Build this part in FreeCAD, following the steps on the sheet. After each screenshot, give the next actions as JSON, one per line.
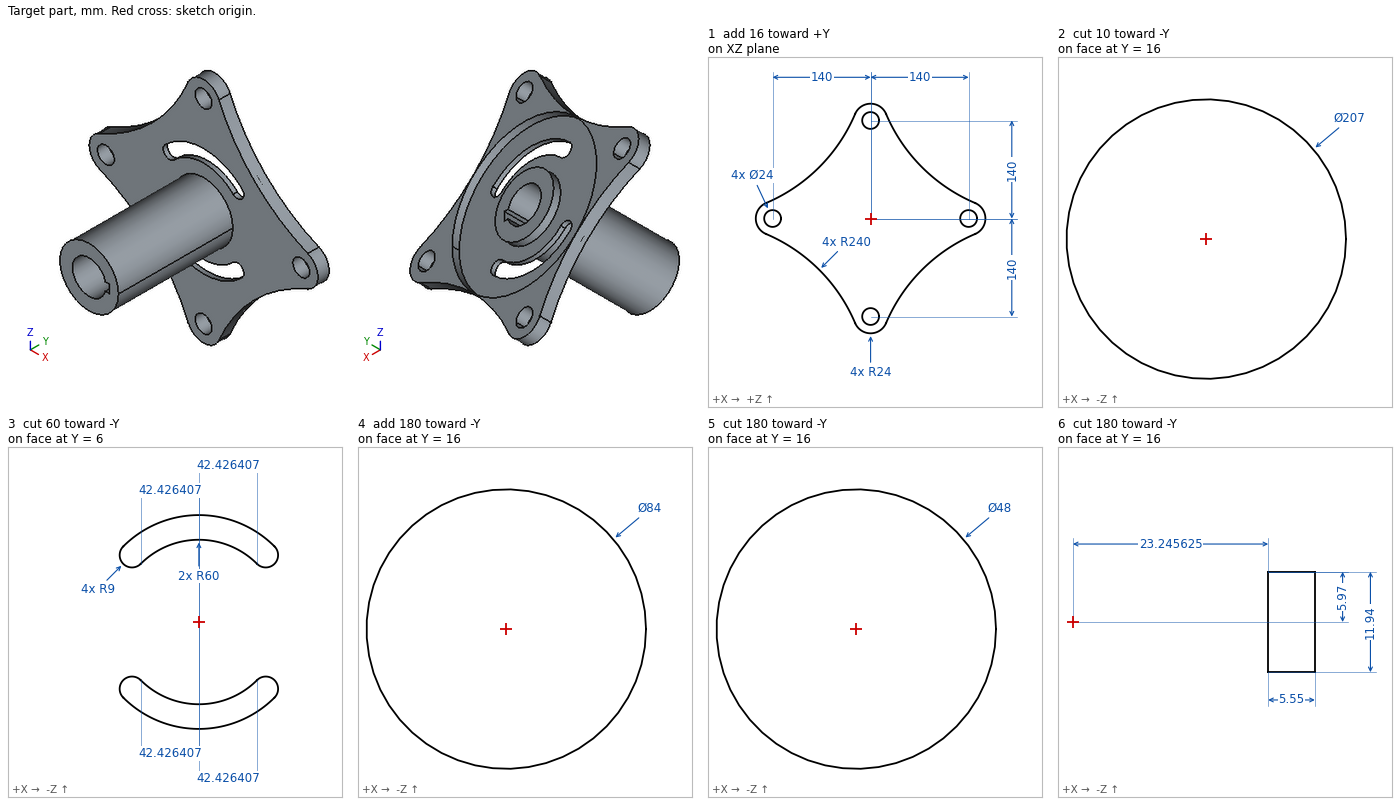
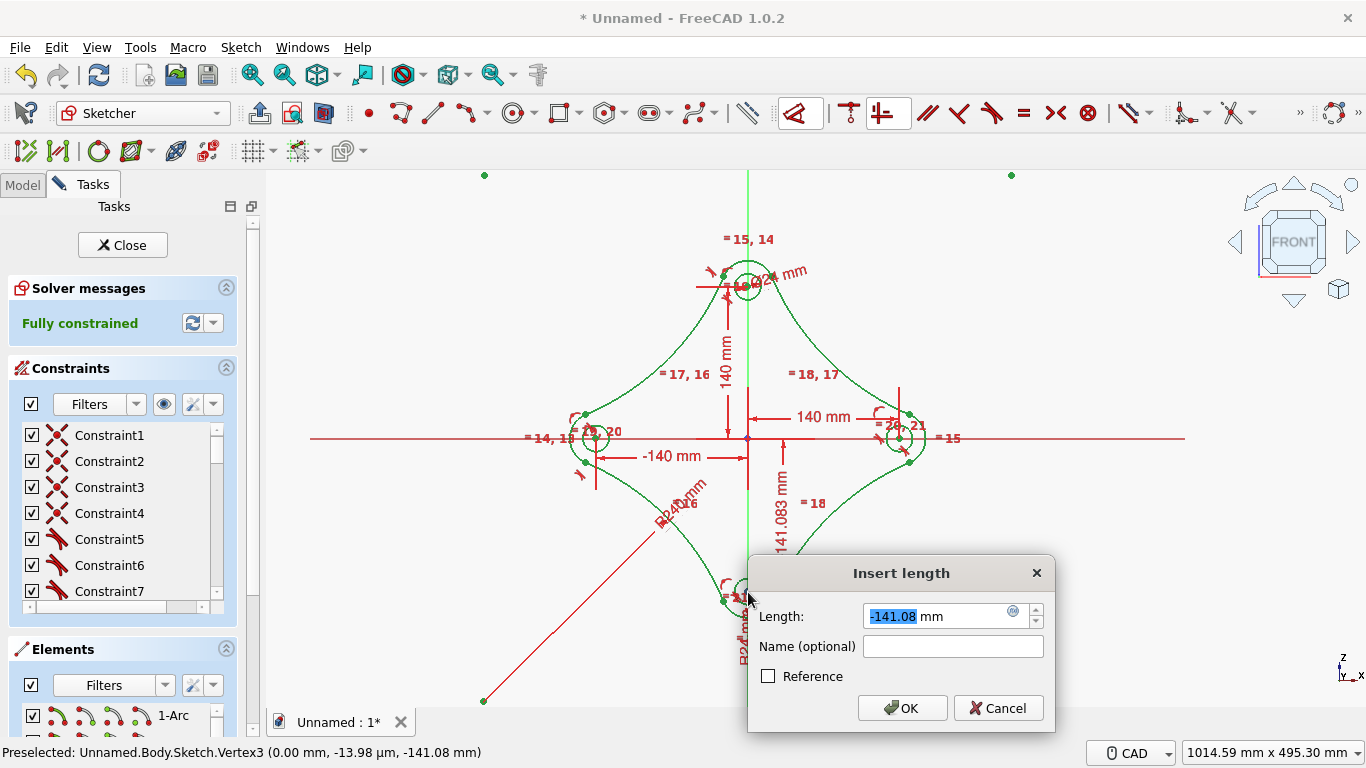
{"action": "type", "text": "-140"}
{"action": "key", "text": "Return"}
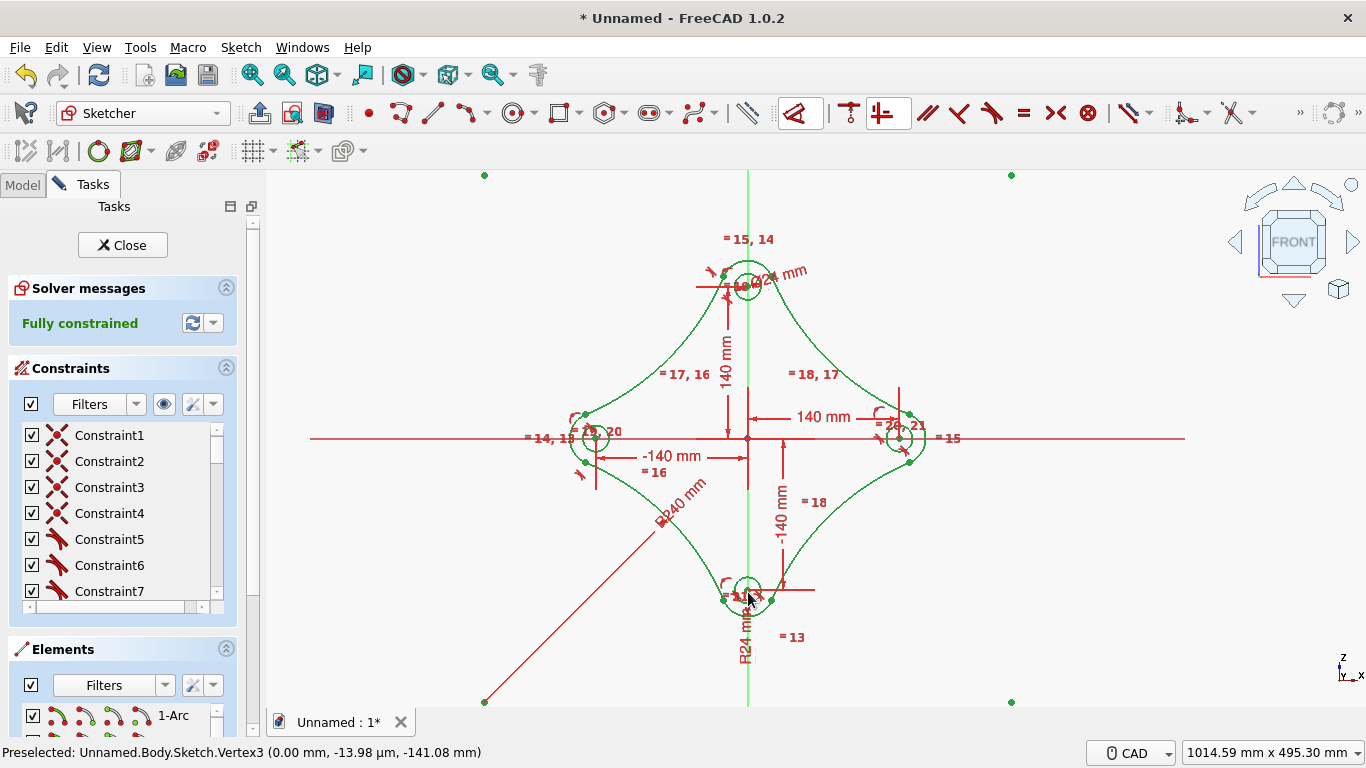
{"action": "left_click", "coordinate": [123, 245]}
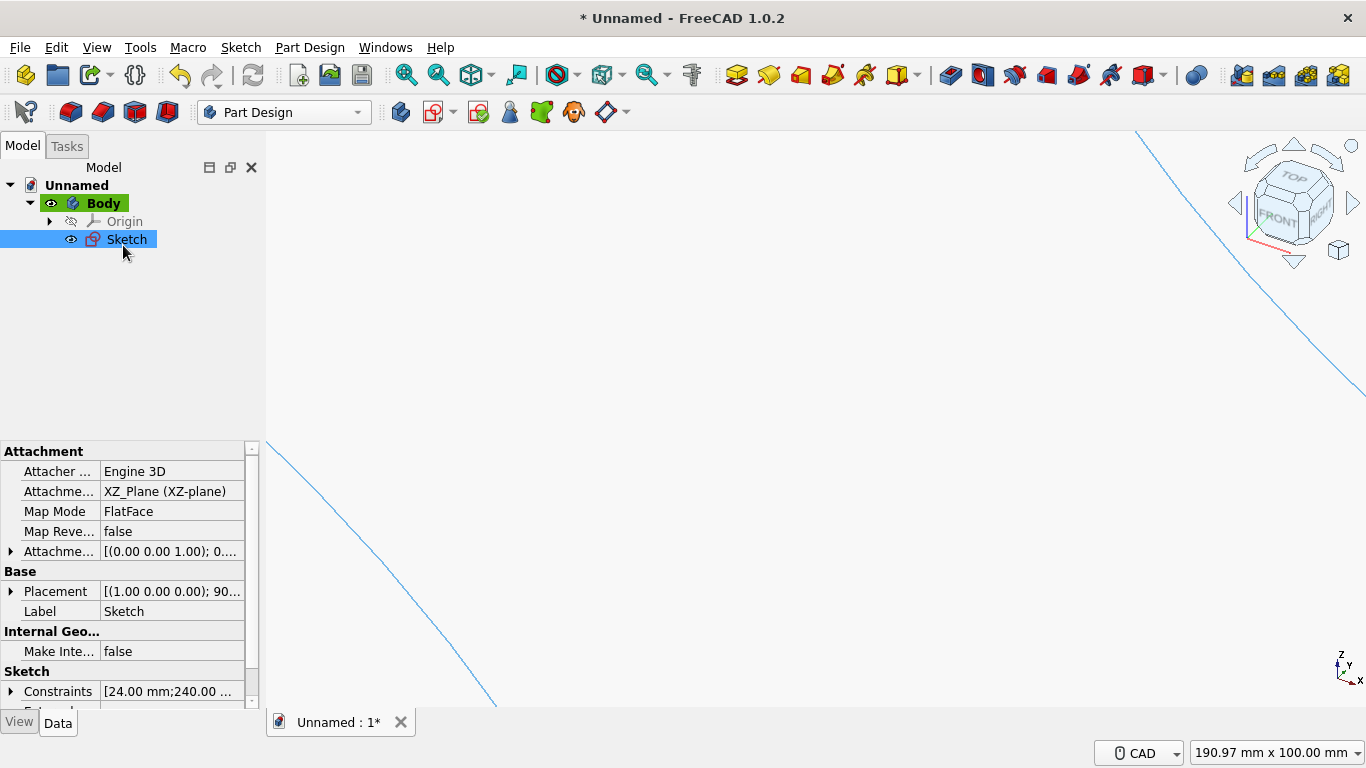
{"action": "left_click", "coordinate": [738, 76]}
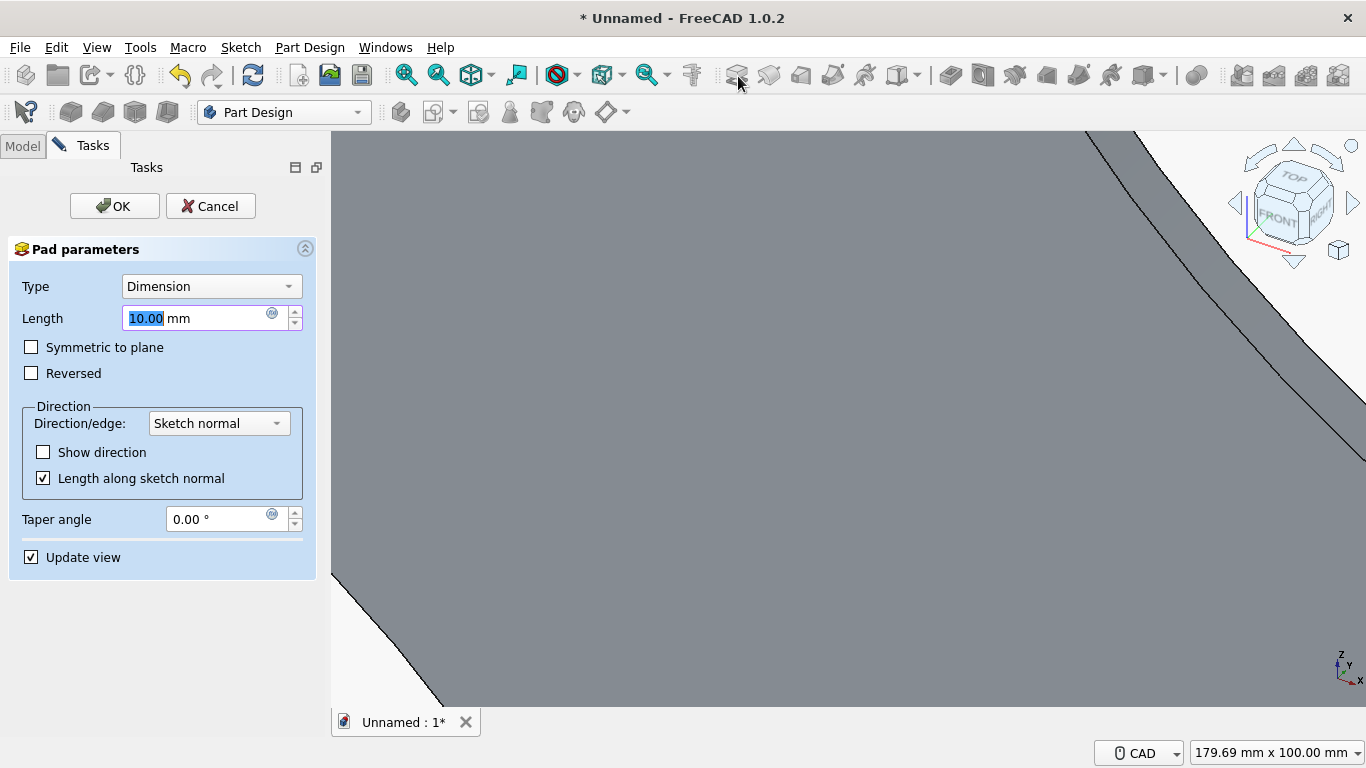
{"action": "type", "text": "16"}
{"action": "key", "text": "Tab"}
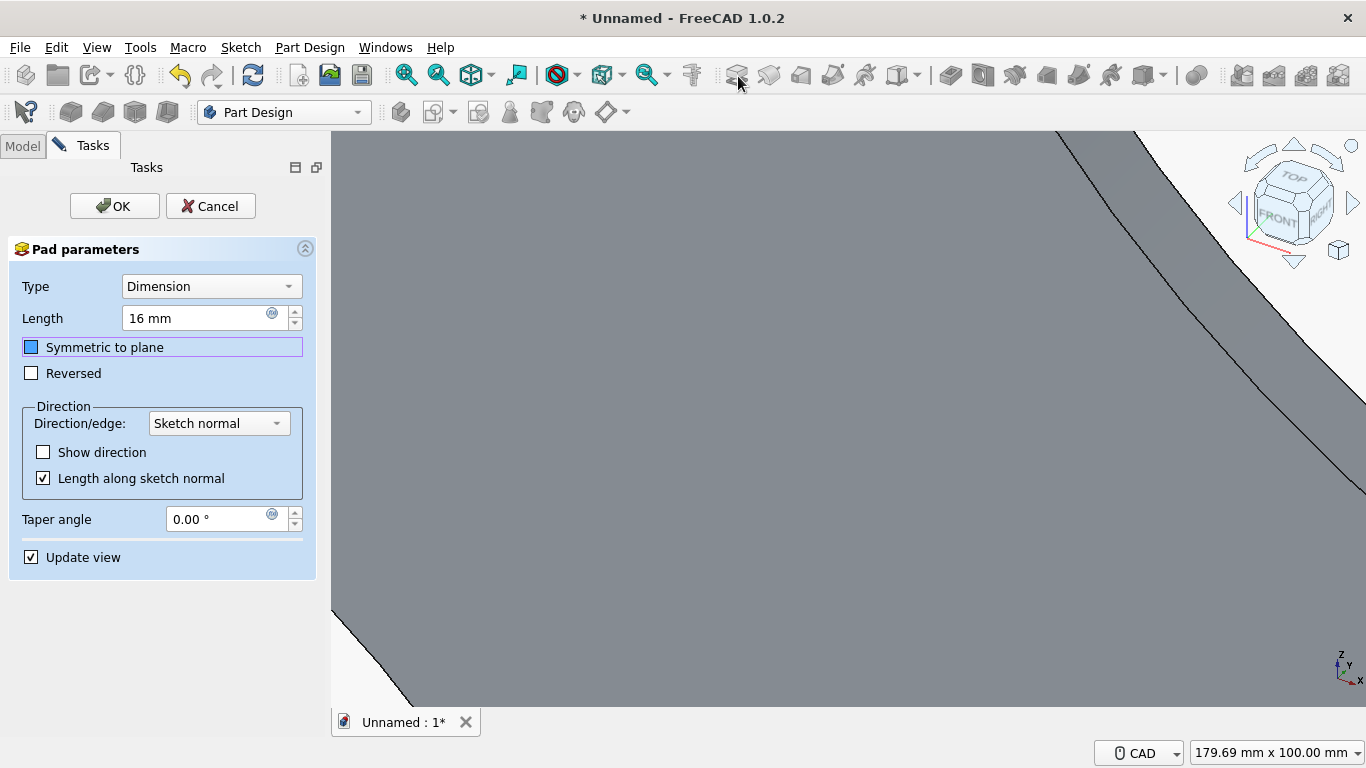
{"action": "left_click", "coordinate": [30, 373]}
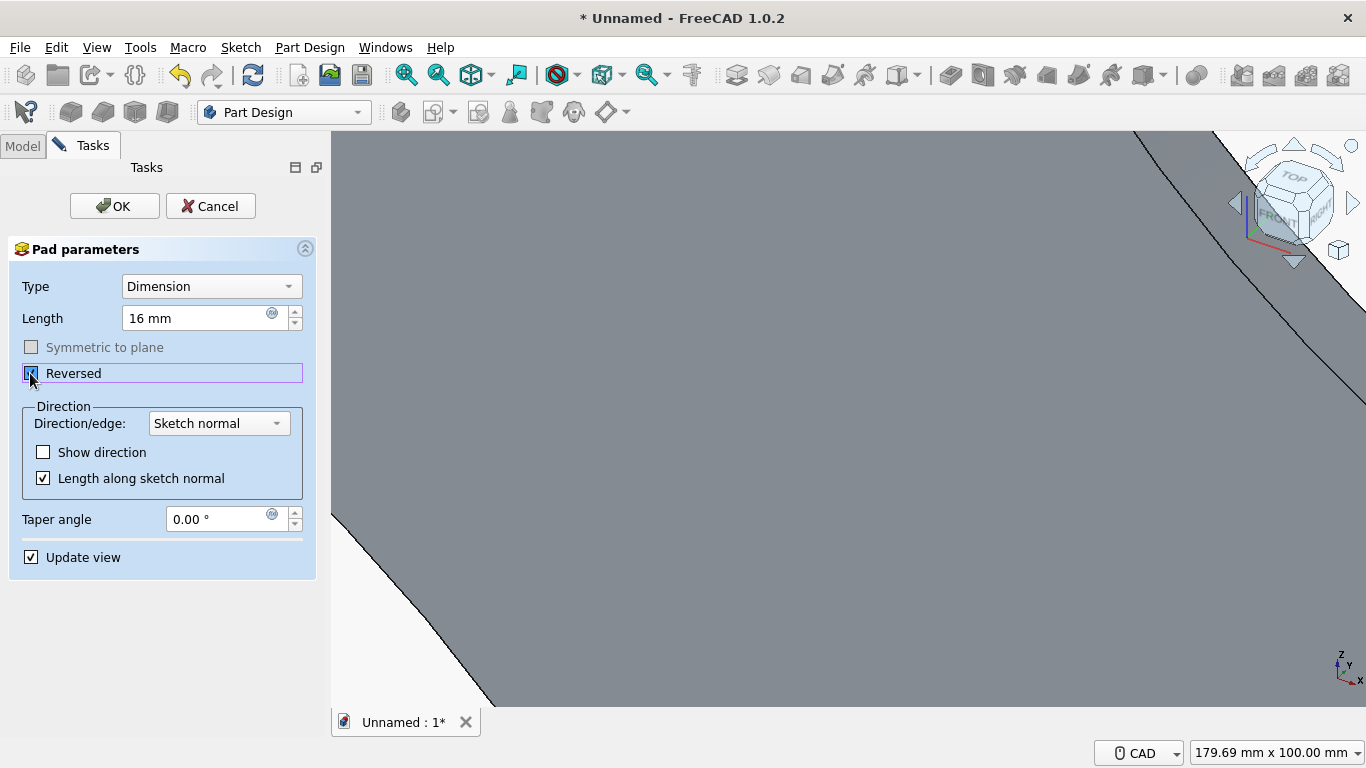
{"action": "left_click", "coordinate": [115, 206]}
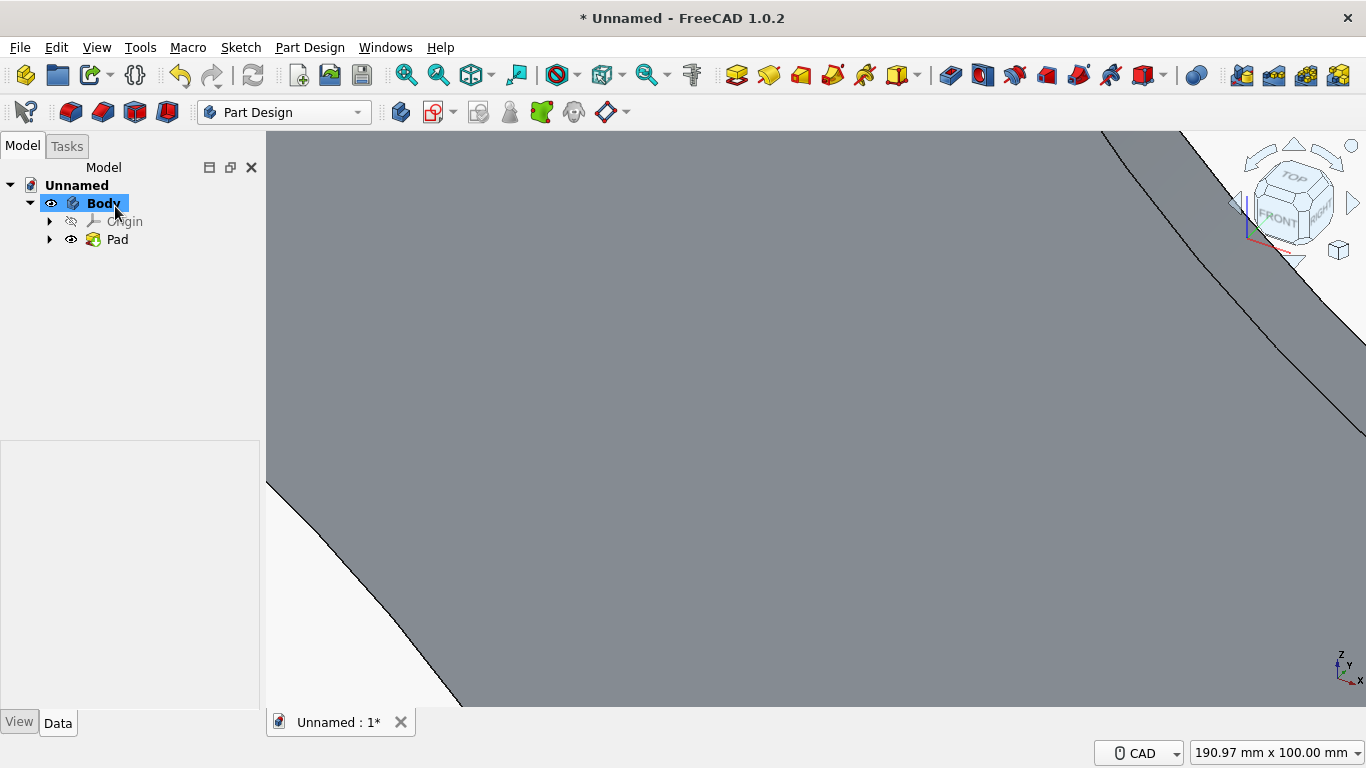
{"action": "left_click", "coordinate": [408, 76]}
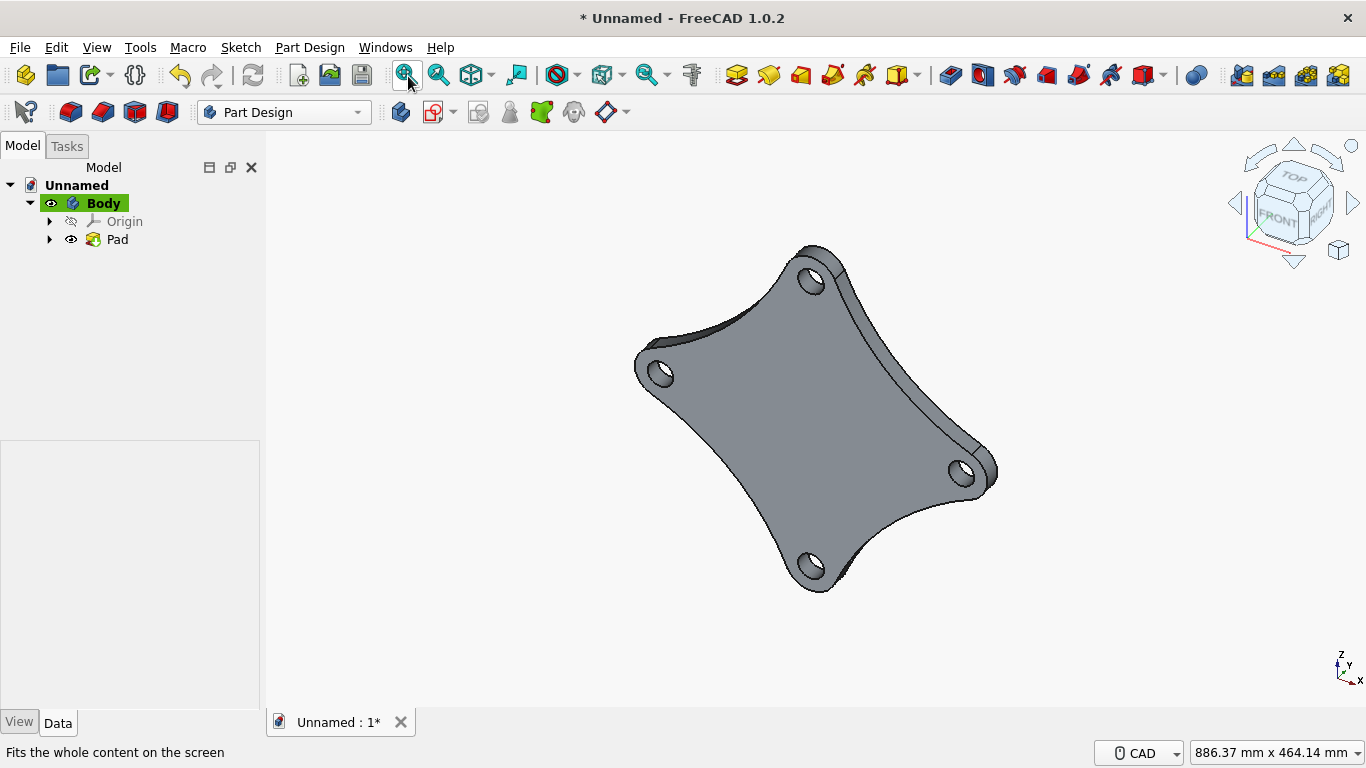
{"action": "key", "text": "4"}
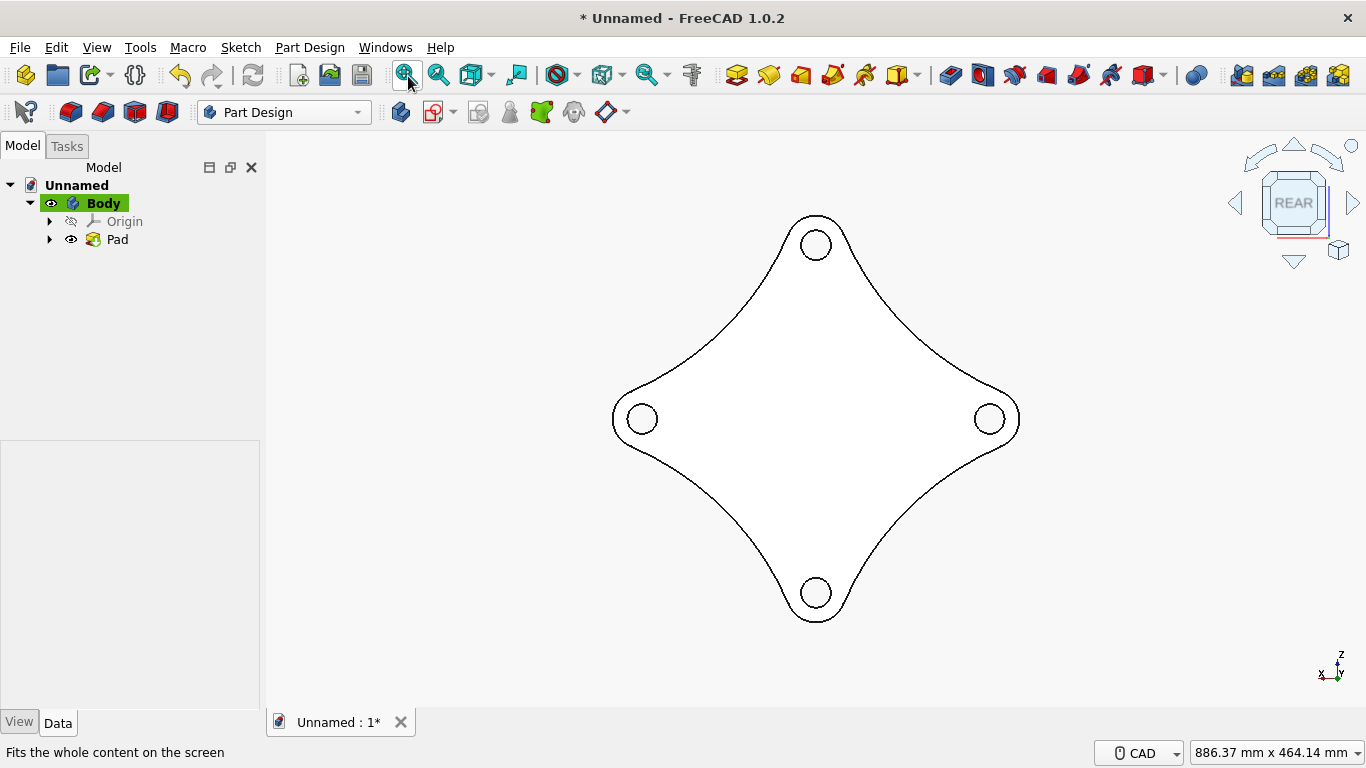
{"action": "left_click", "coordinate": [816, 418]}